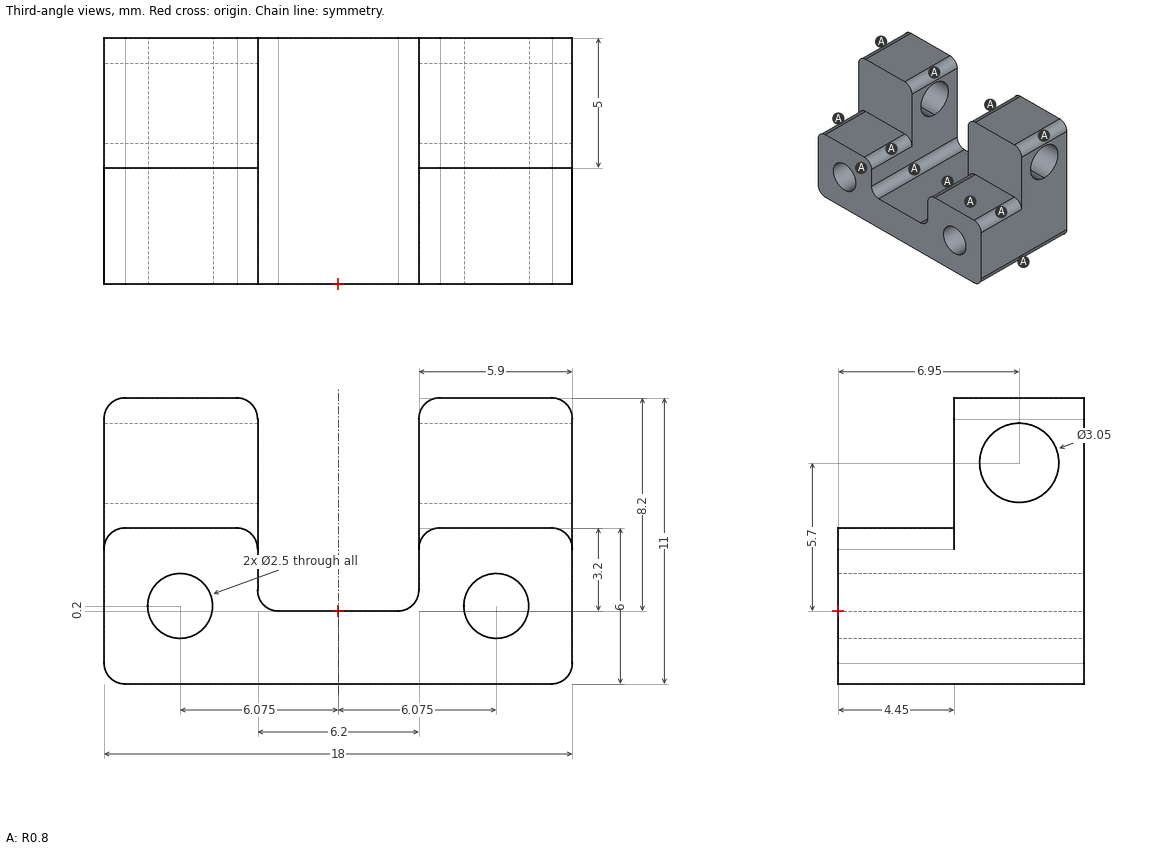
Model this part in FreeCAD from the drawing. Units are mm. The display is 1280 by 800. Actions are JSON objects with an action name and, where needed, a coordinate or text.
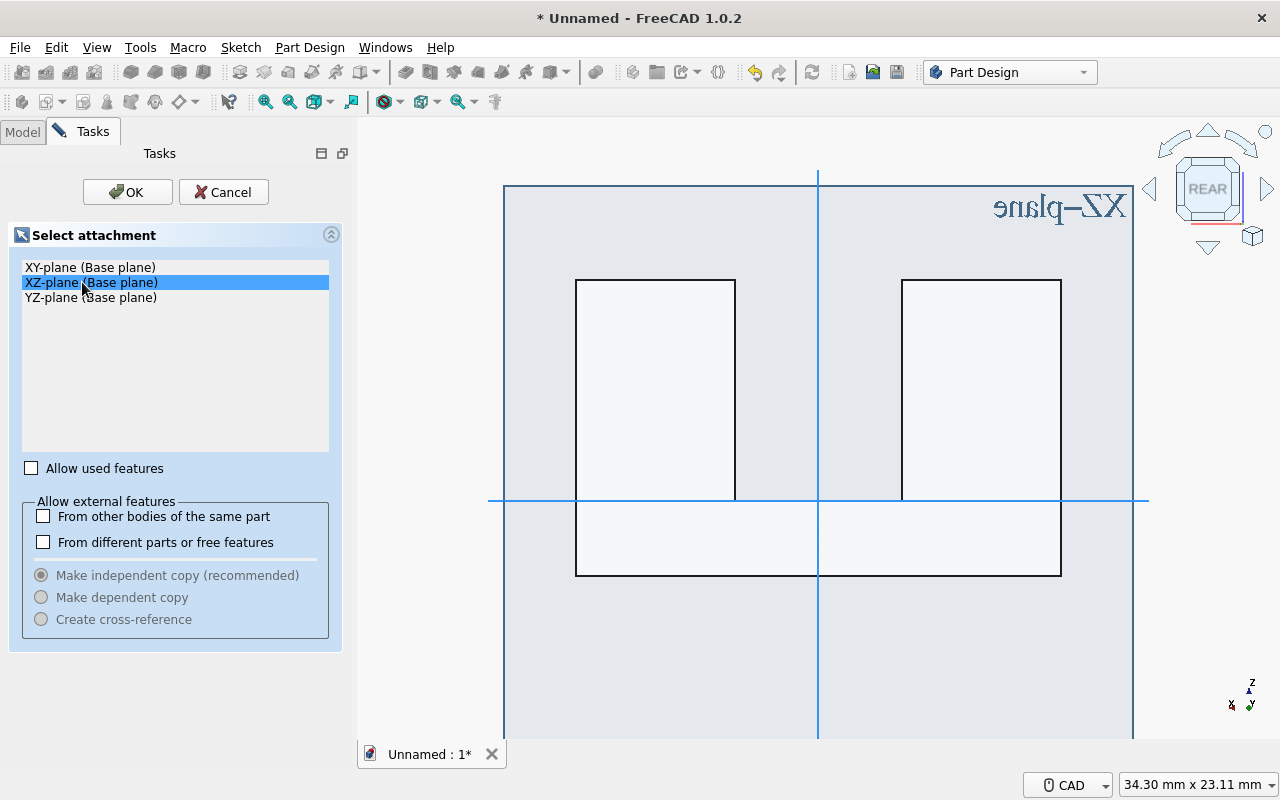
{"action": "left_click", "coordinate": [128, 192]}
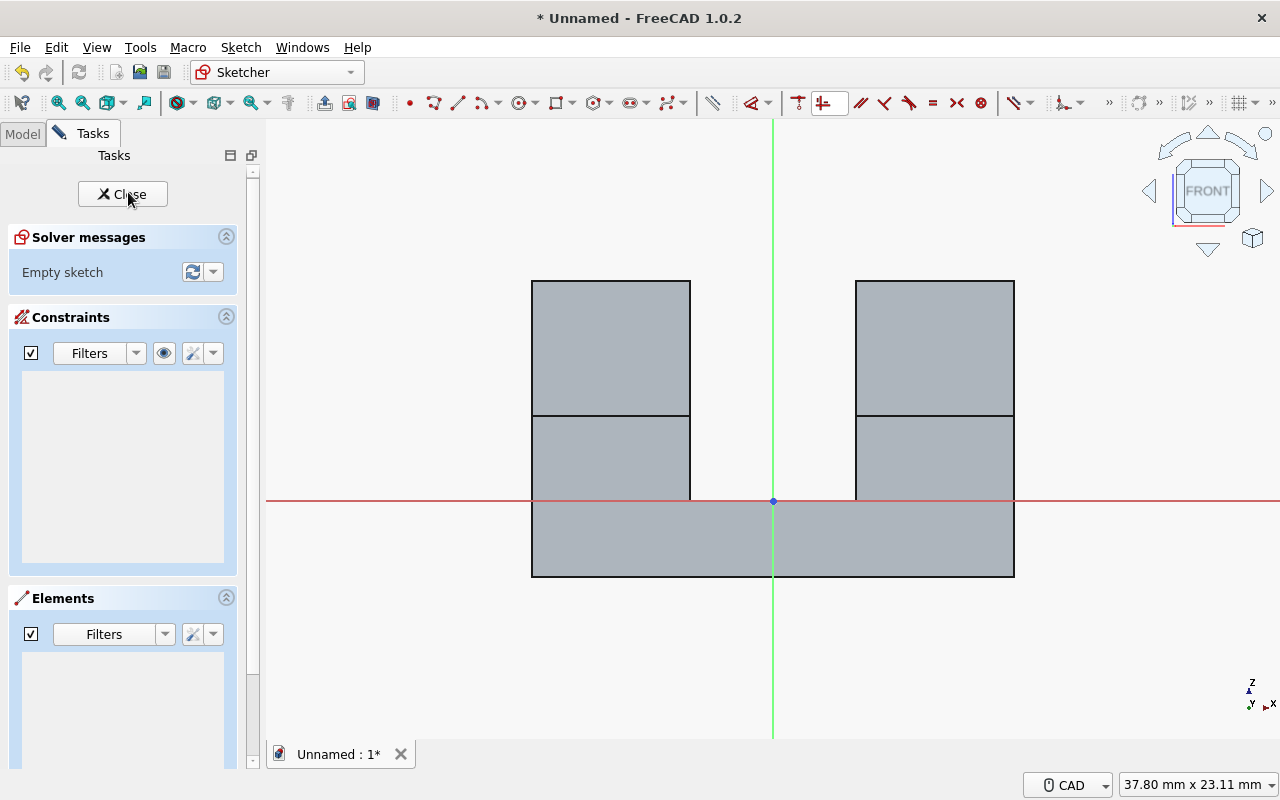
{"action": "scroll", "coordinate": [912, 632], "scroll_direction": "up", "scroll_amount": 2}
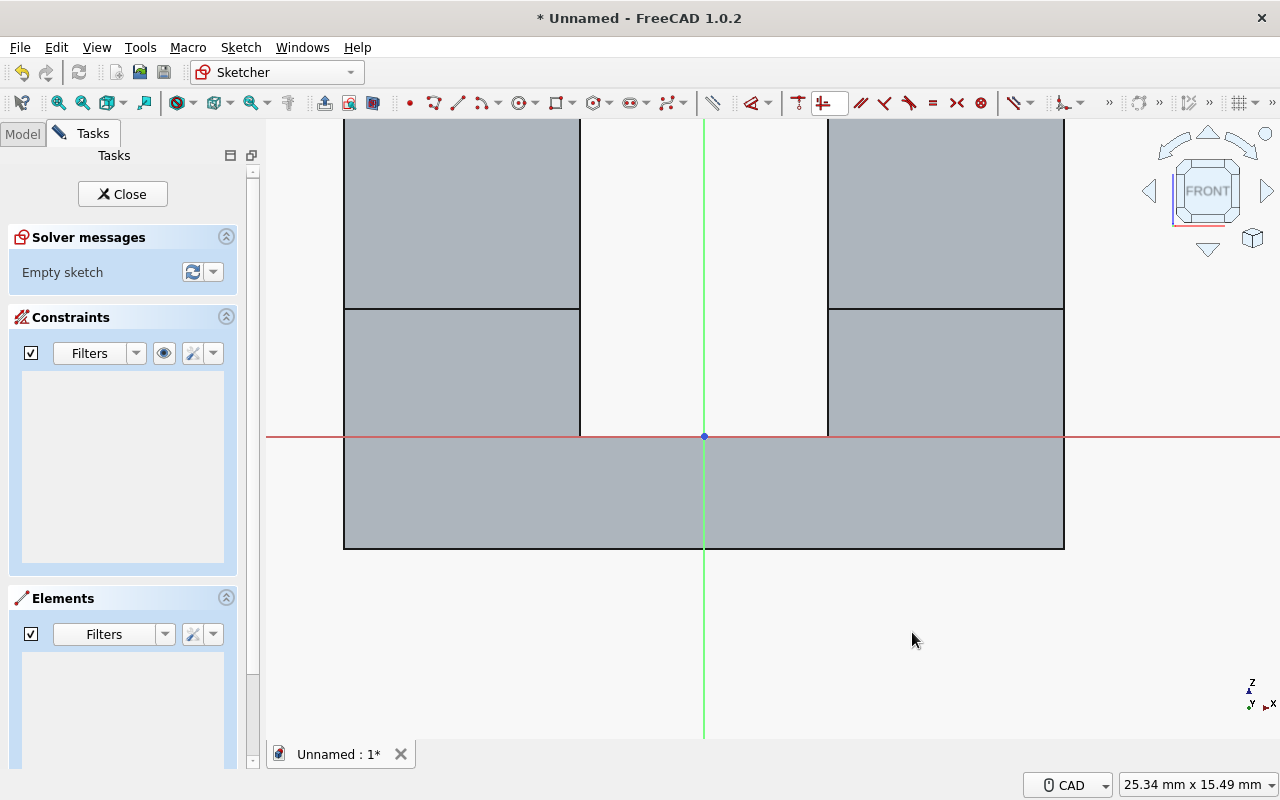
{"action": "left_click", "coordinate": [520, 104]}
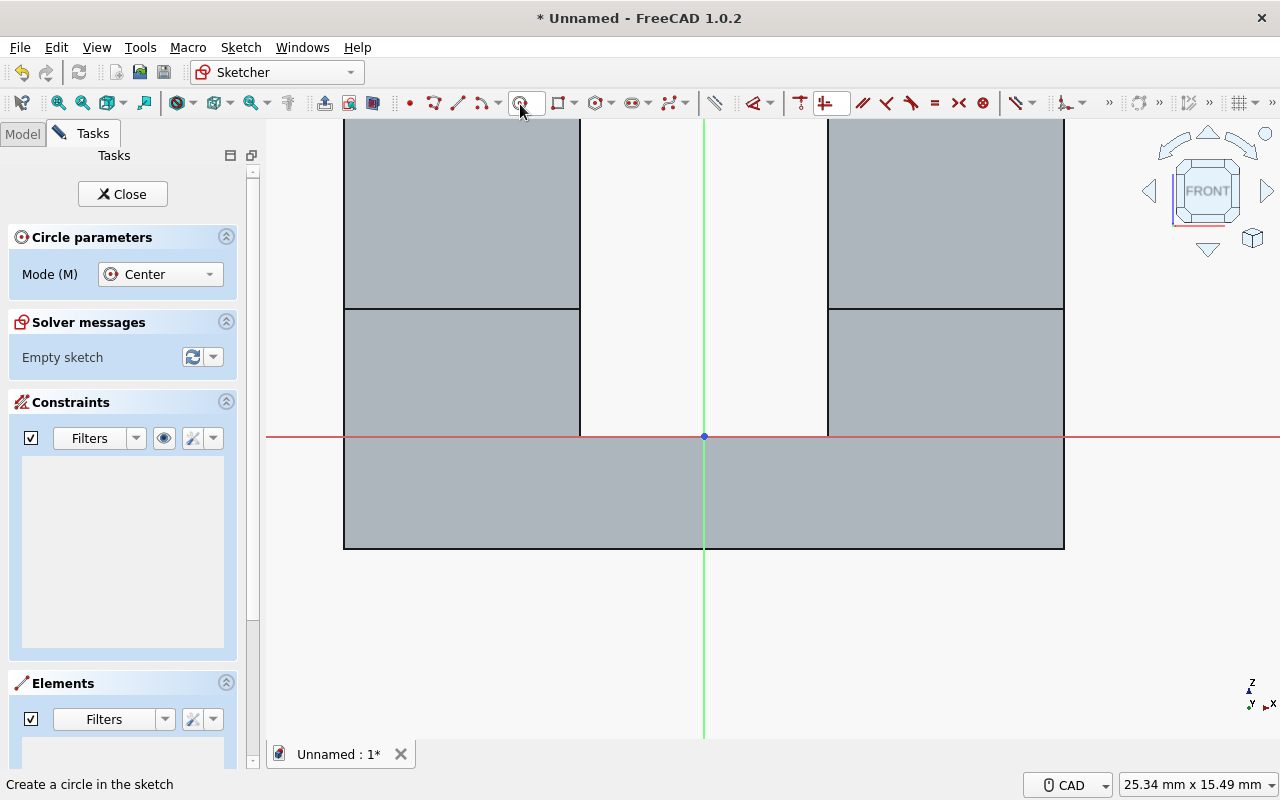
{"action": "scroll", "coordinate": [461, 429], "scroll_direction": "up", "scroll_amount": 4}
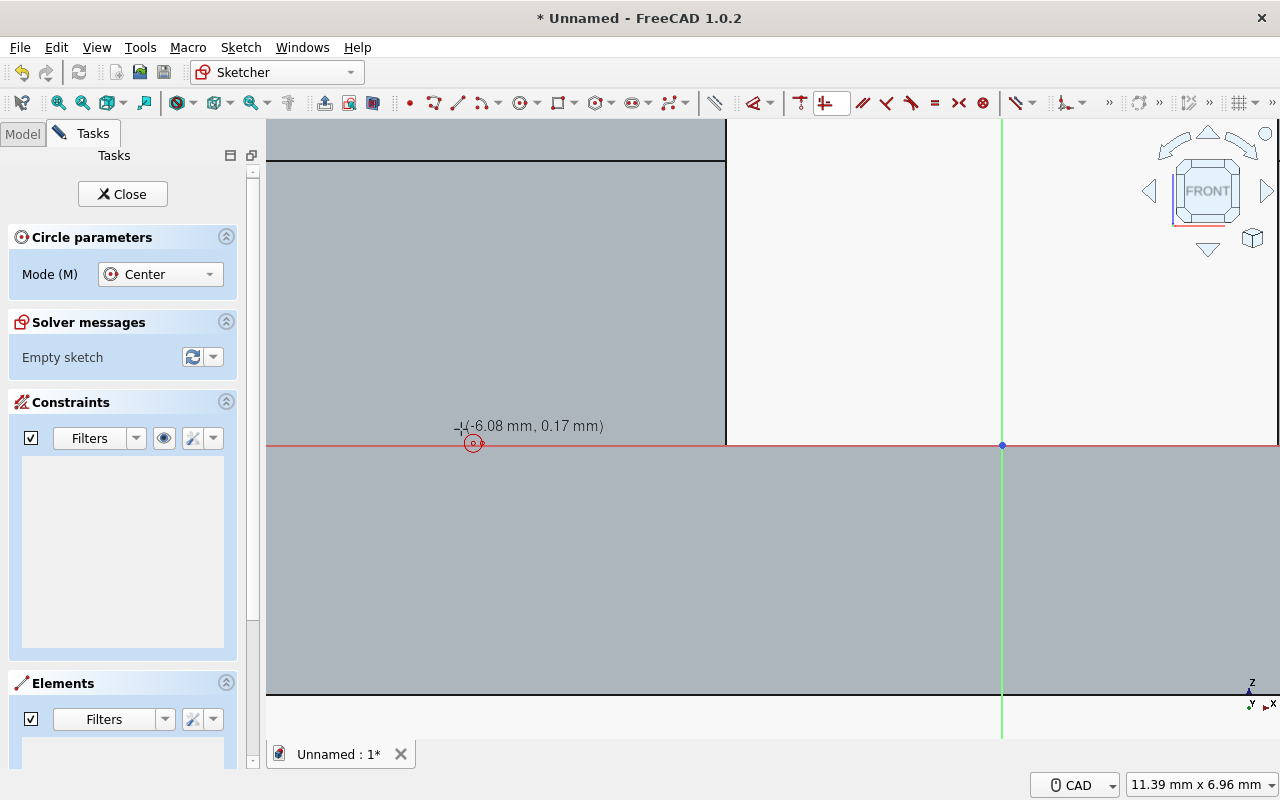
{"action": "left_click", "coordinate": [461, 428]}
{"action": "mouse_move", "coordinate": [540, 349]}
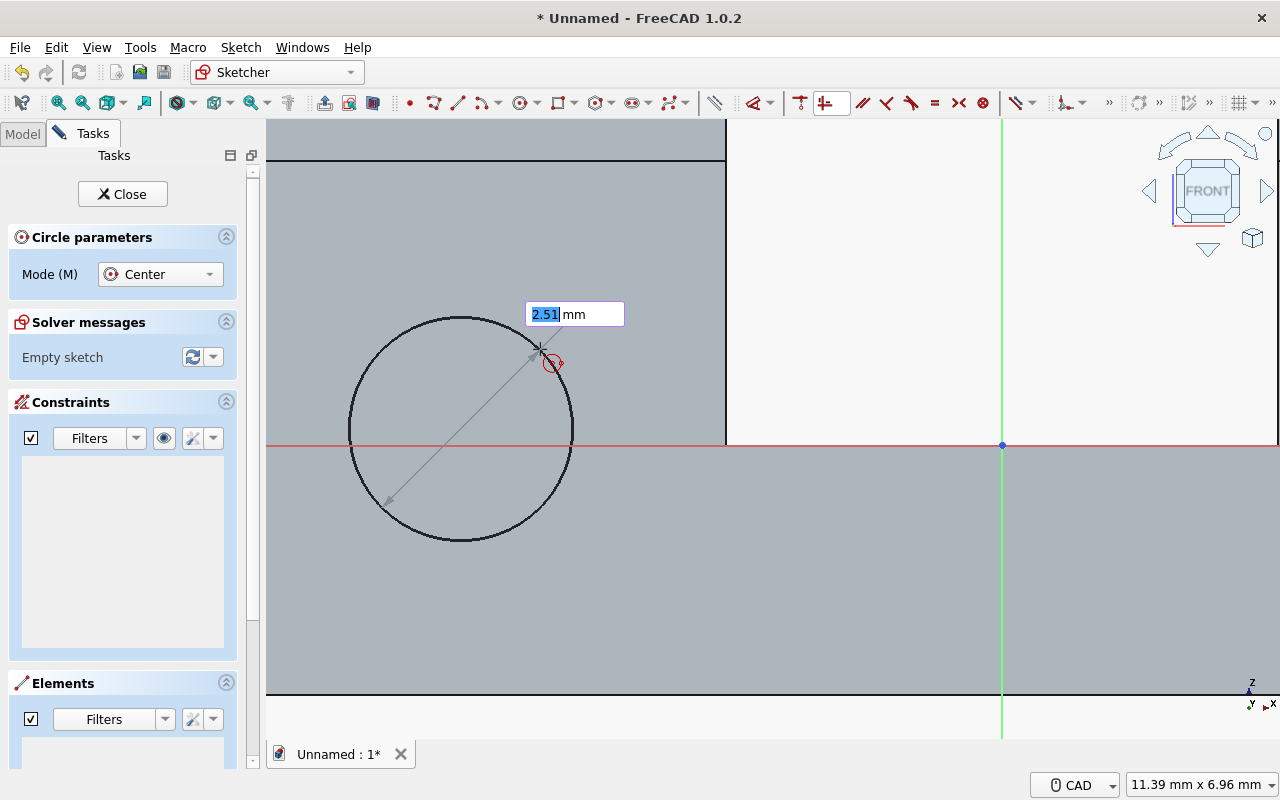
{"action": "type", "text": "2.5"}
{"action": "key", "text": "Return"}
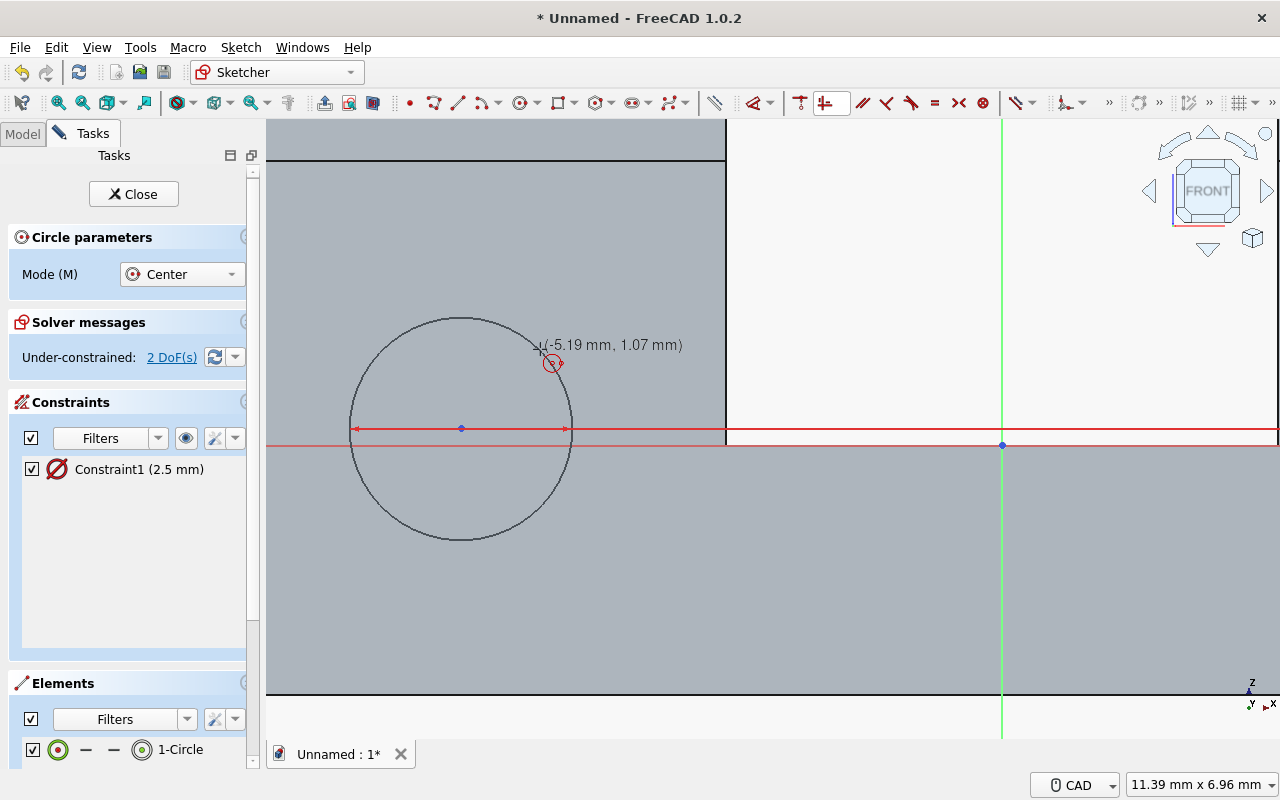
{"action": "scroll", "coordinate": [462, 430], "scroll_direction": "down", "scroll_amount": 4}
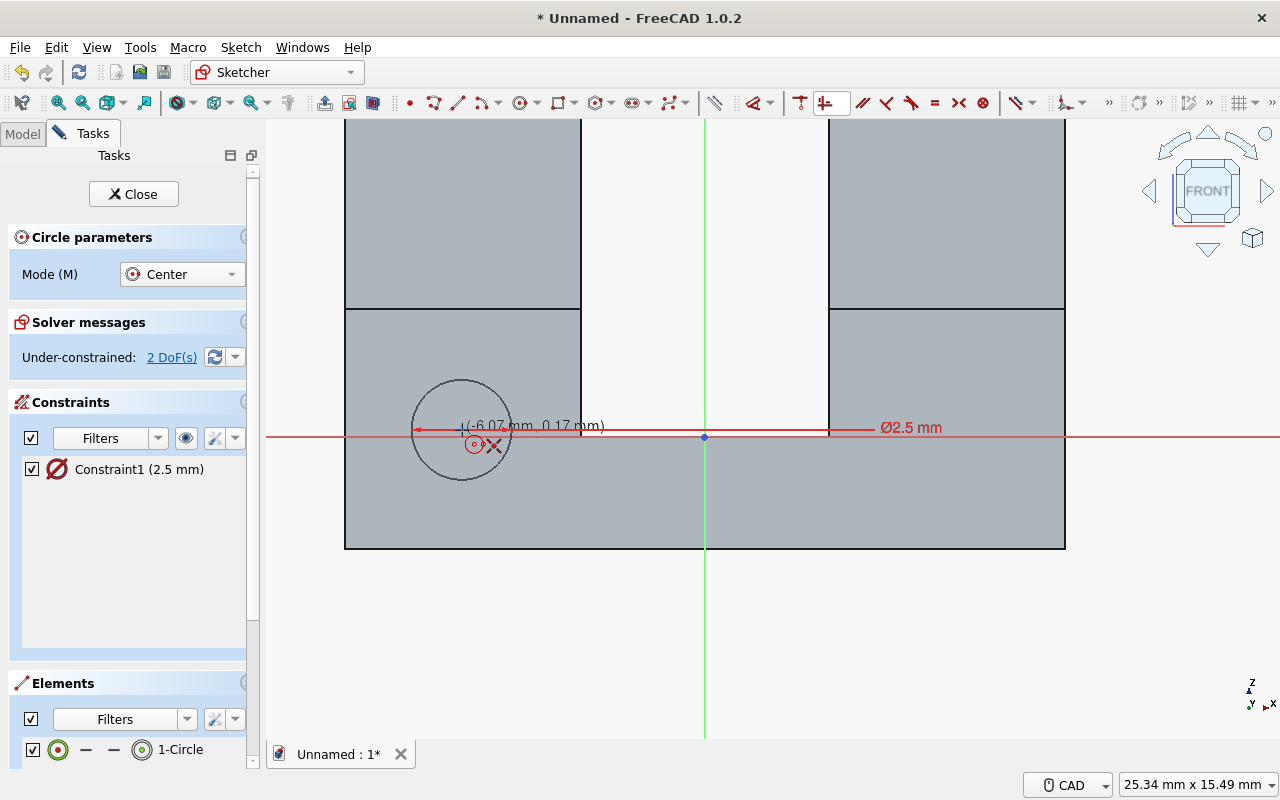
{"action": "scroll", "coordinate": [948, 429], "scroll_direction": "up", "scroll_amount": 4}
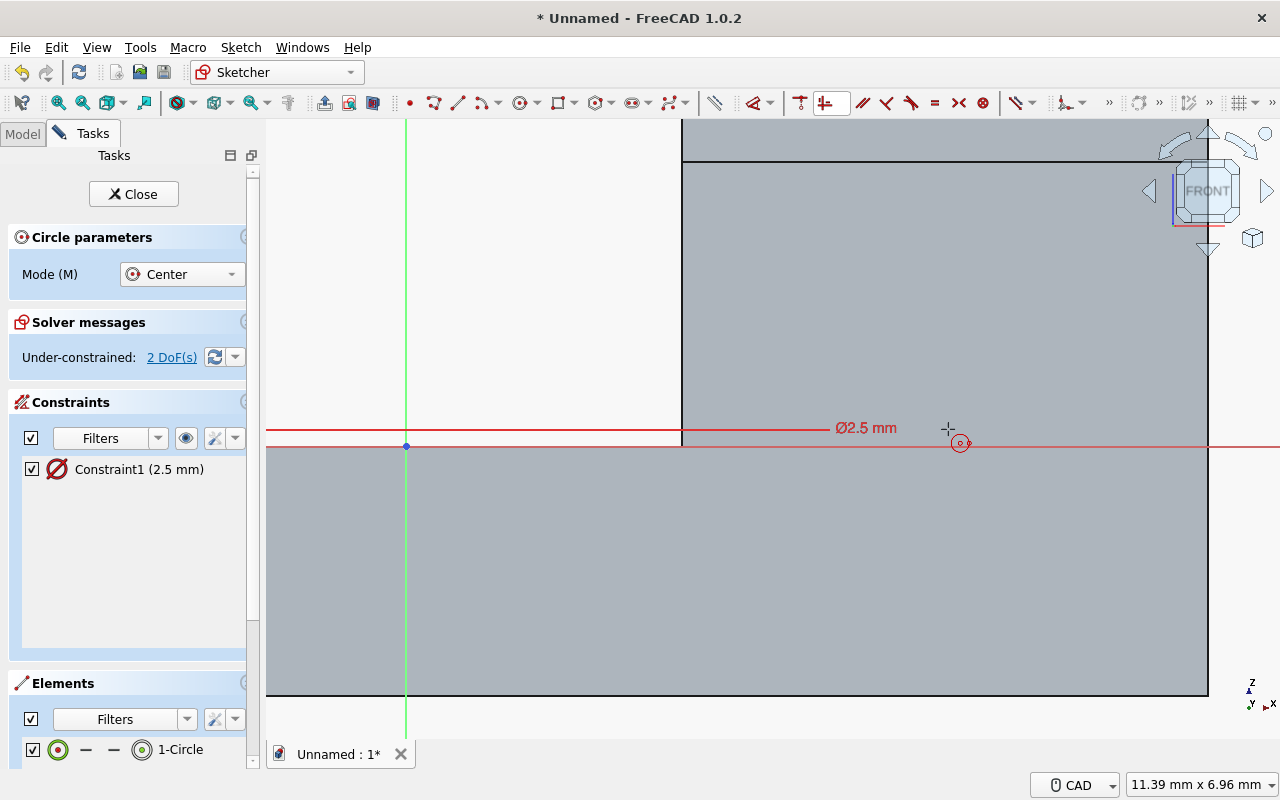
{"action": "left_click", "coordinate": [947, 429]}
{"action": "mouse_move", "coordinate": [1026, 350]}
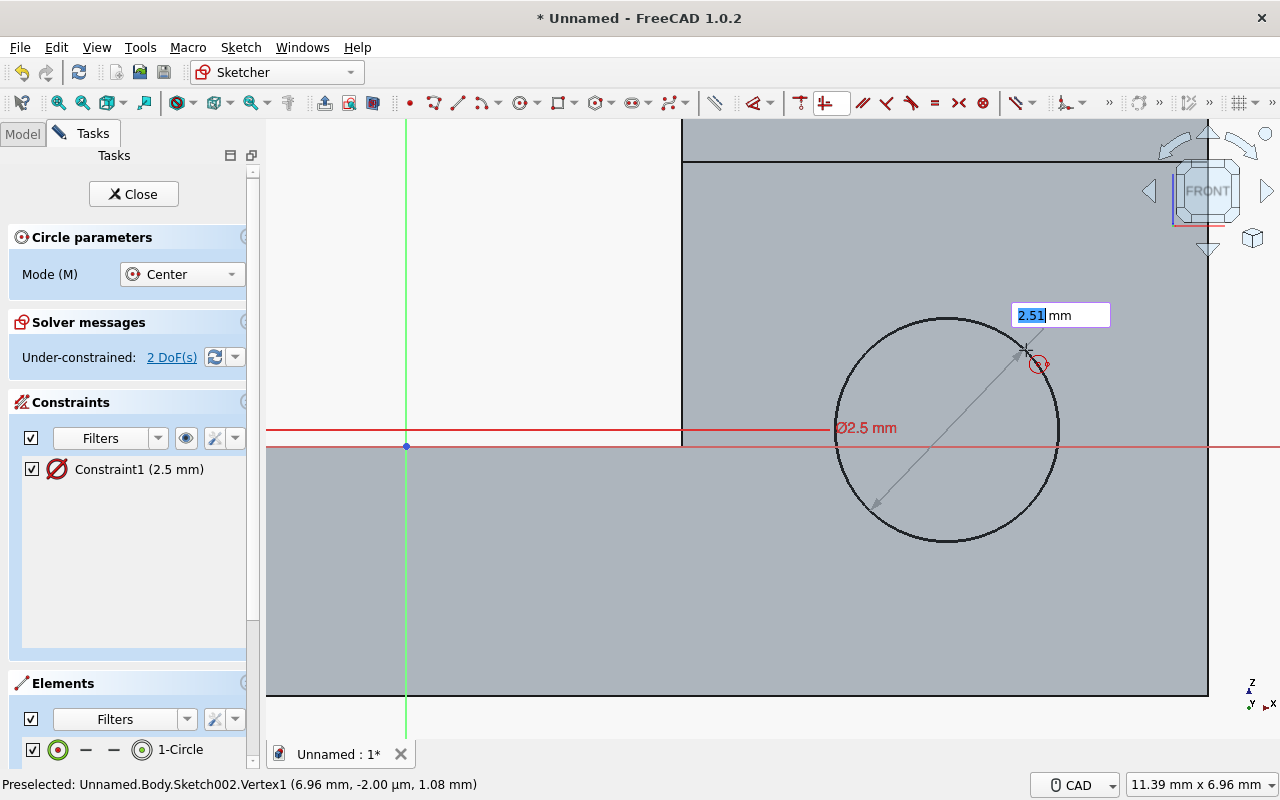
{"action": "type", "text": "2.5"}
{"action": "key", "text": "Return"}
{"action": "key", "text": "Escape"}